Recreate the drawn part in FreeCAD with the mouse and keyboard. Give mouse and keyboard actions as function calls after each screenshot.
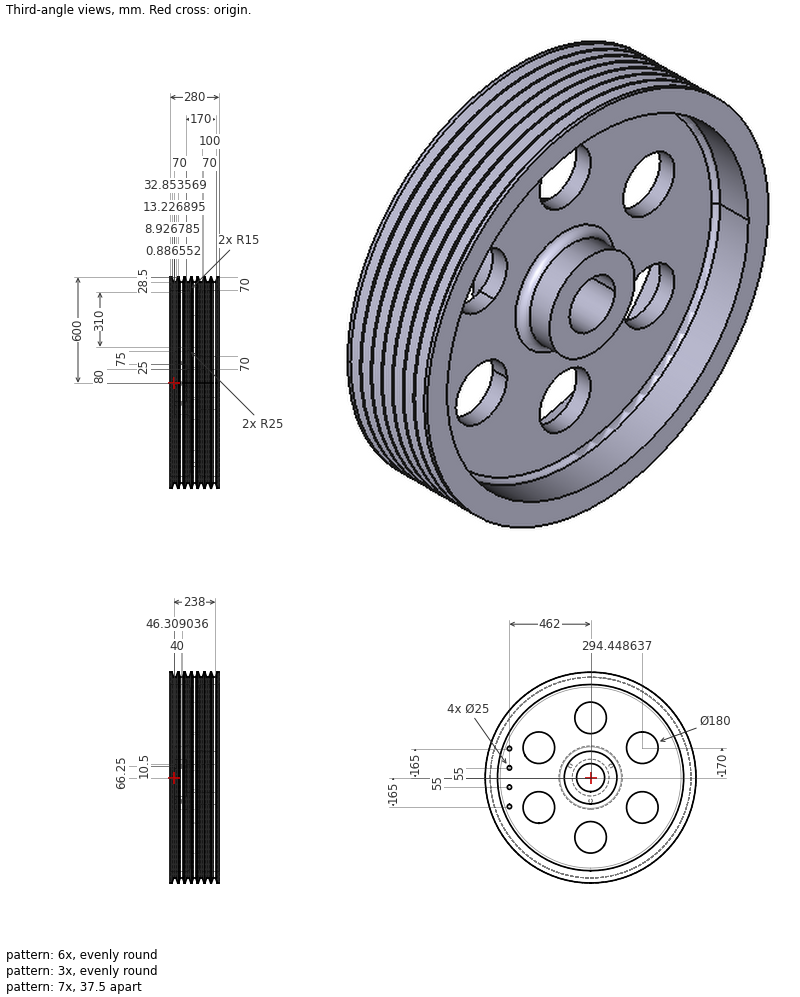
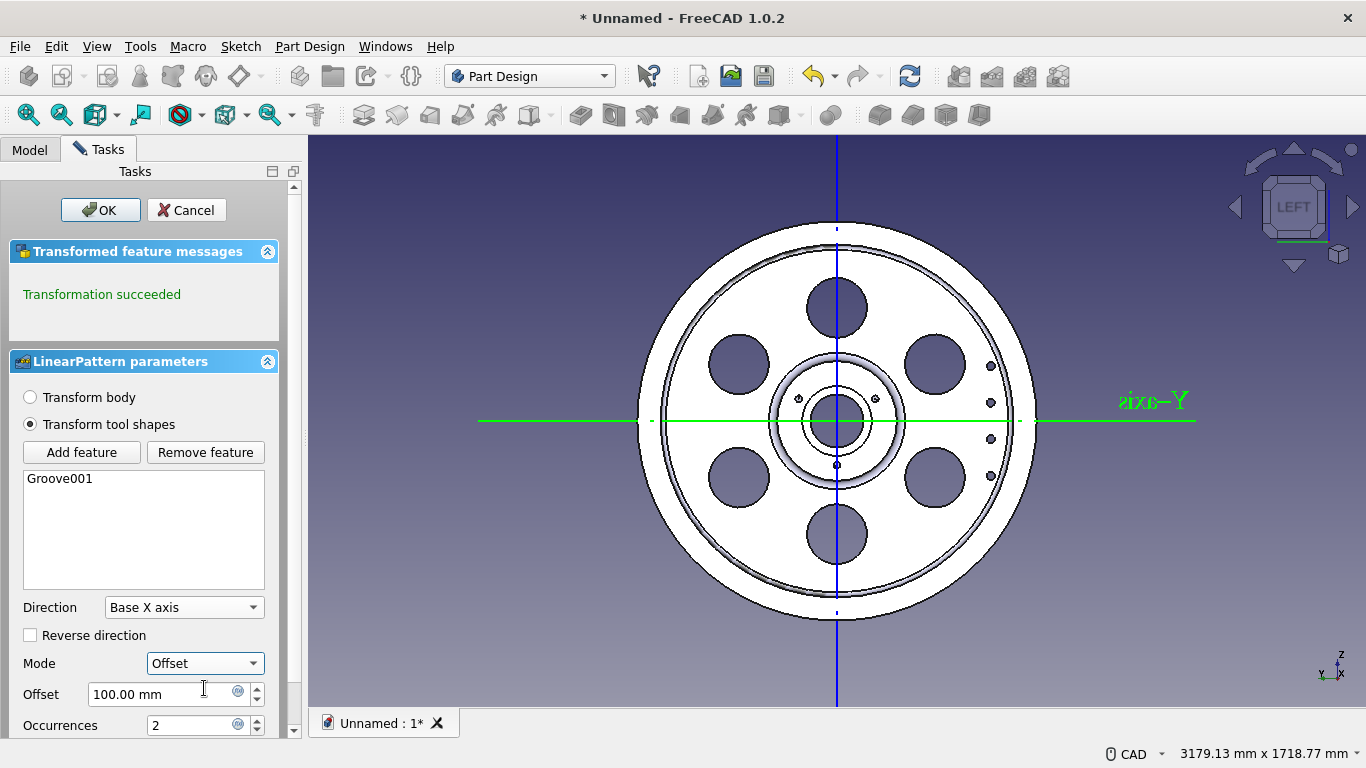
triple_click(170, 694)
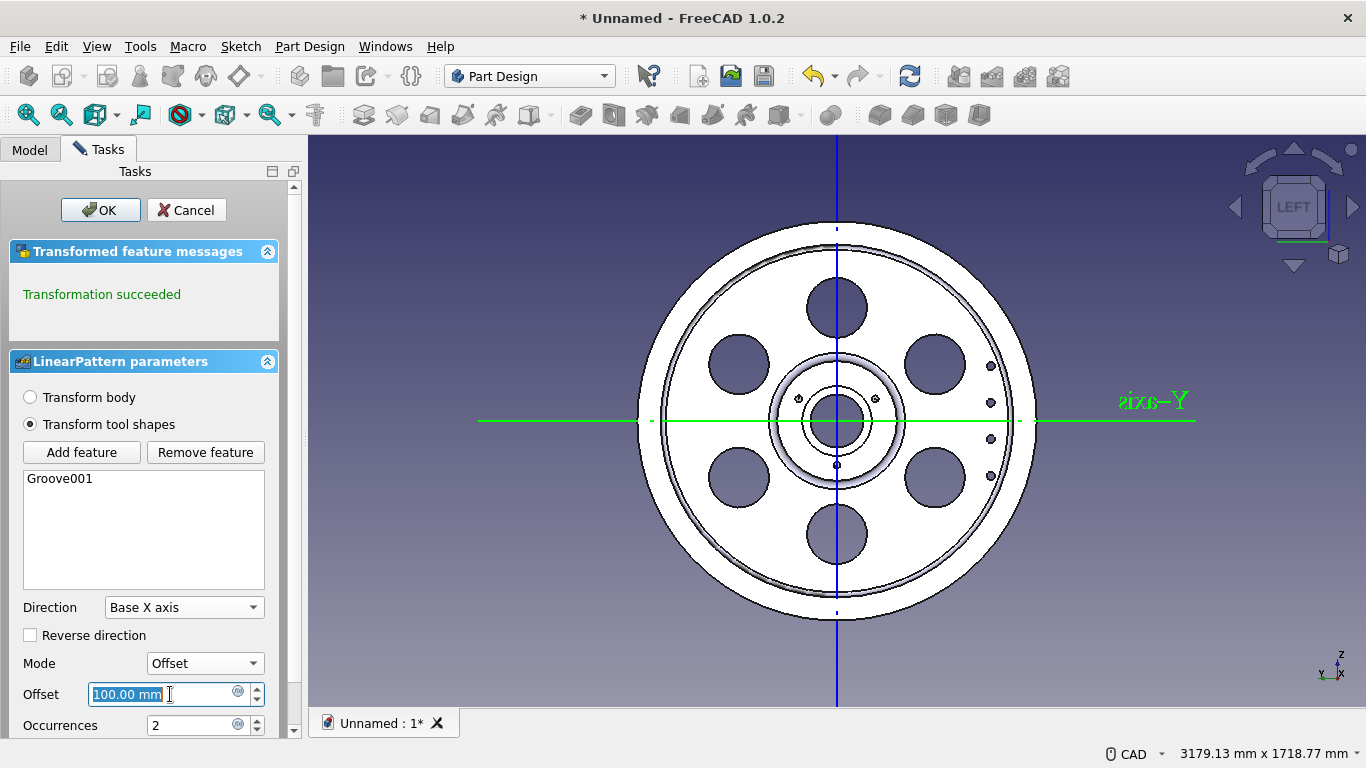
text(37.5)
key(Tab)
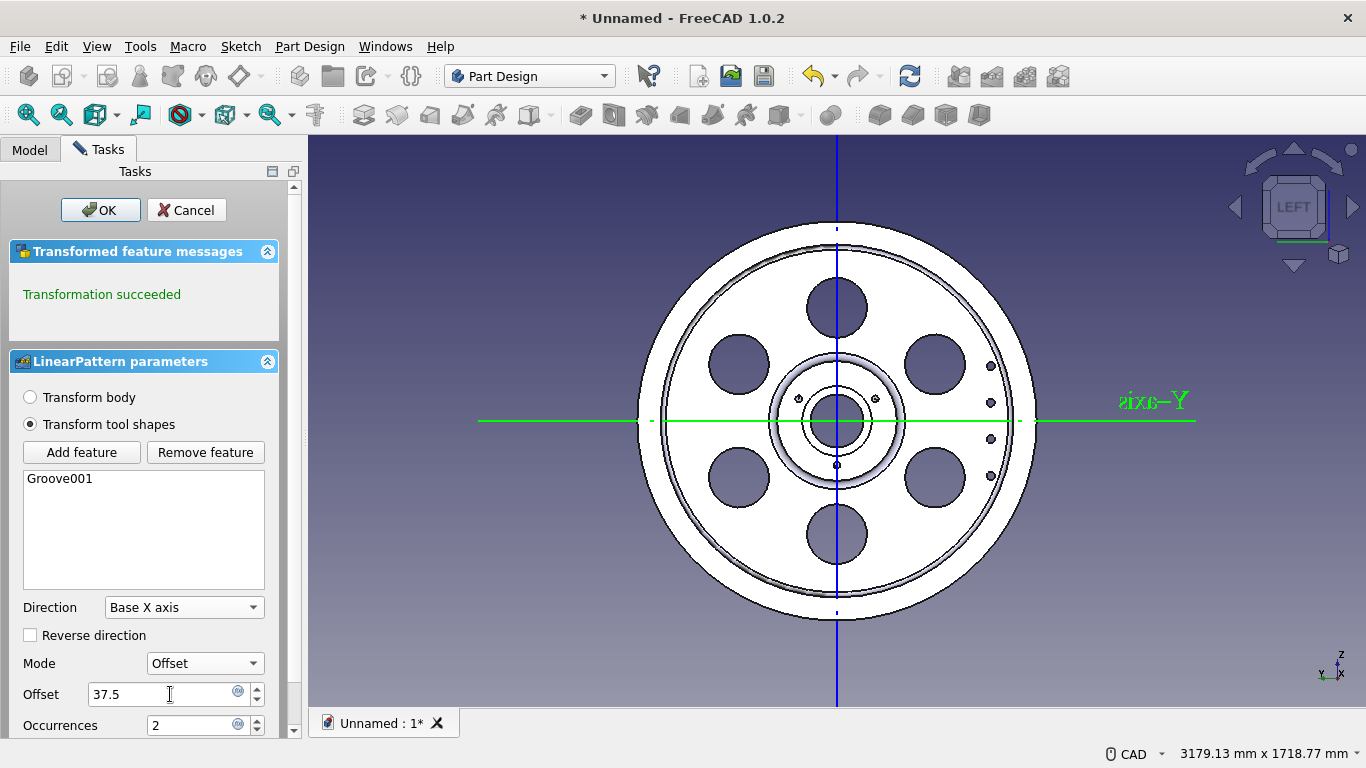
triple_click(199, 726)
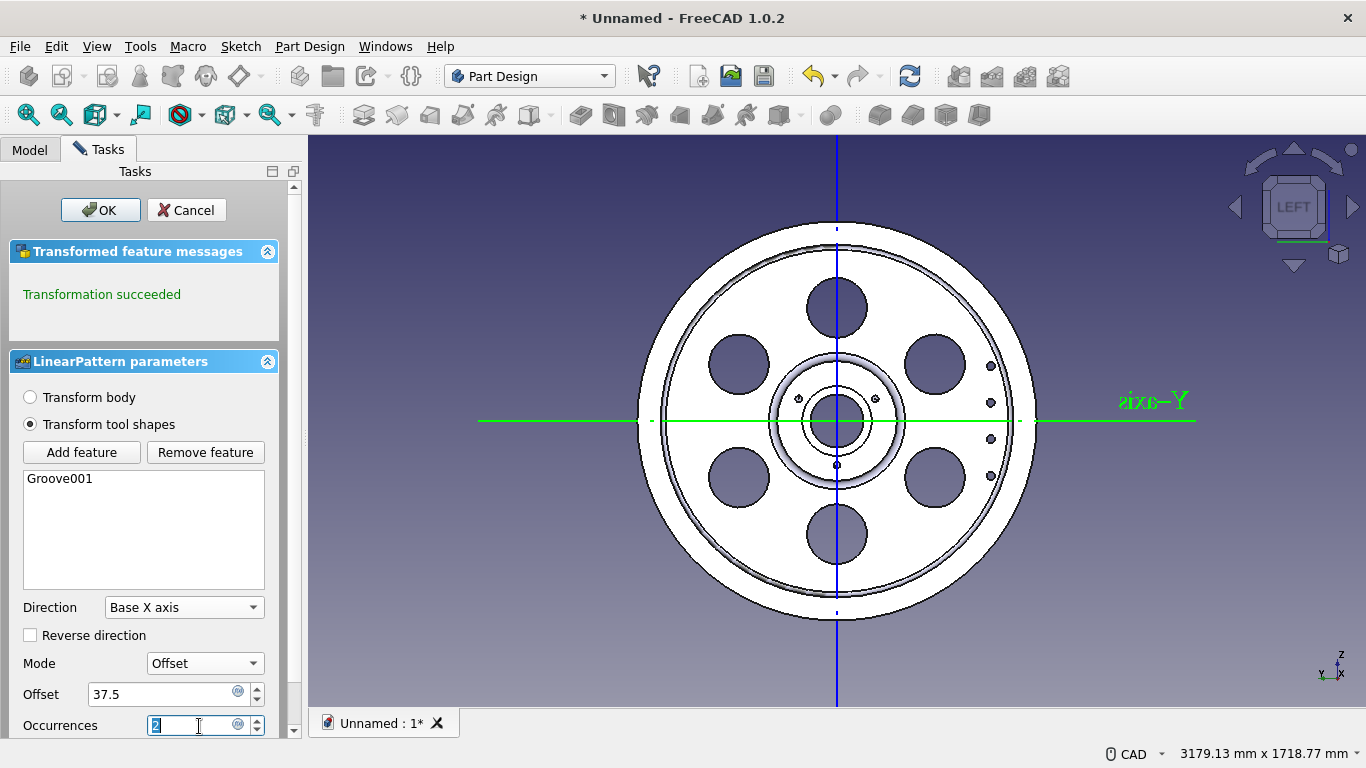
text(7)
key(Tab)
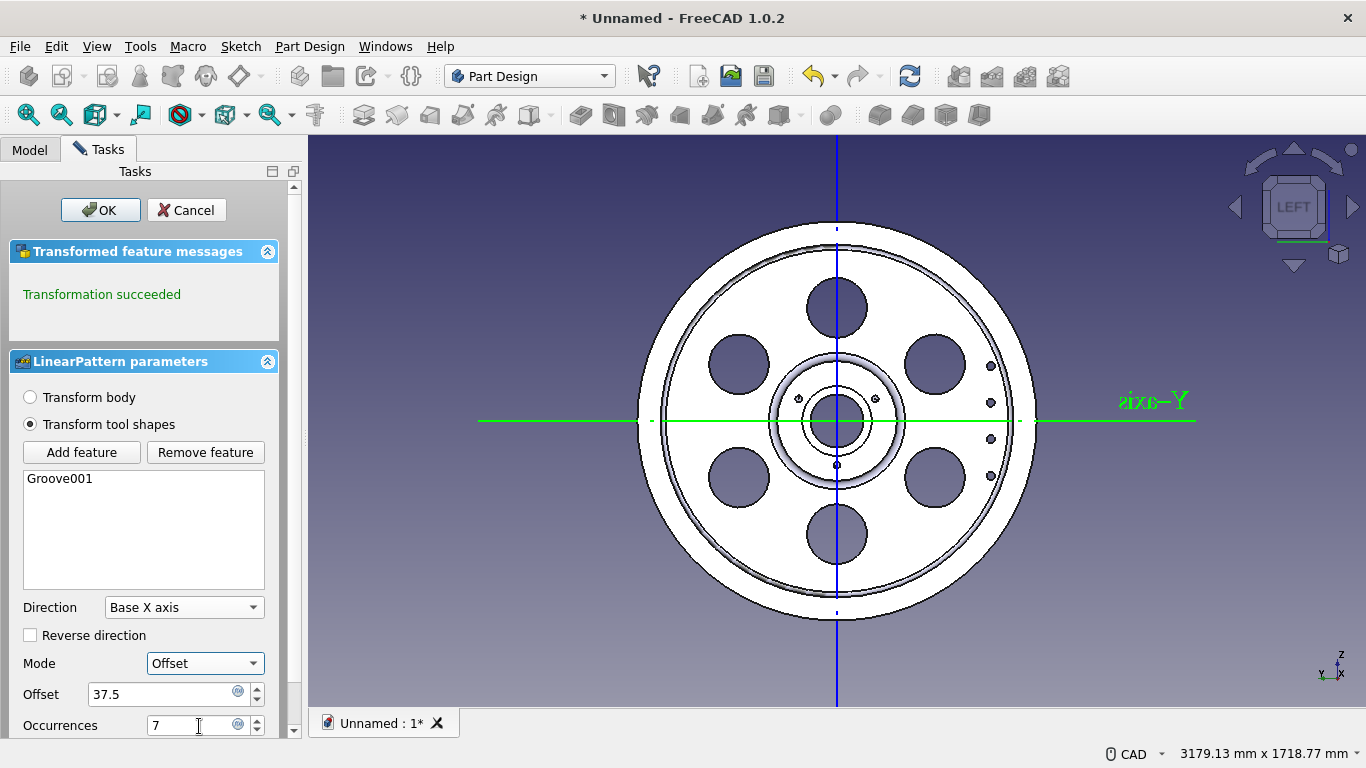
click(101, 210)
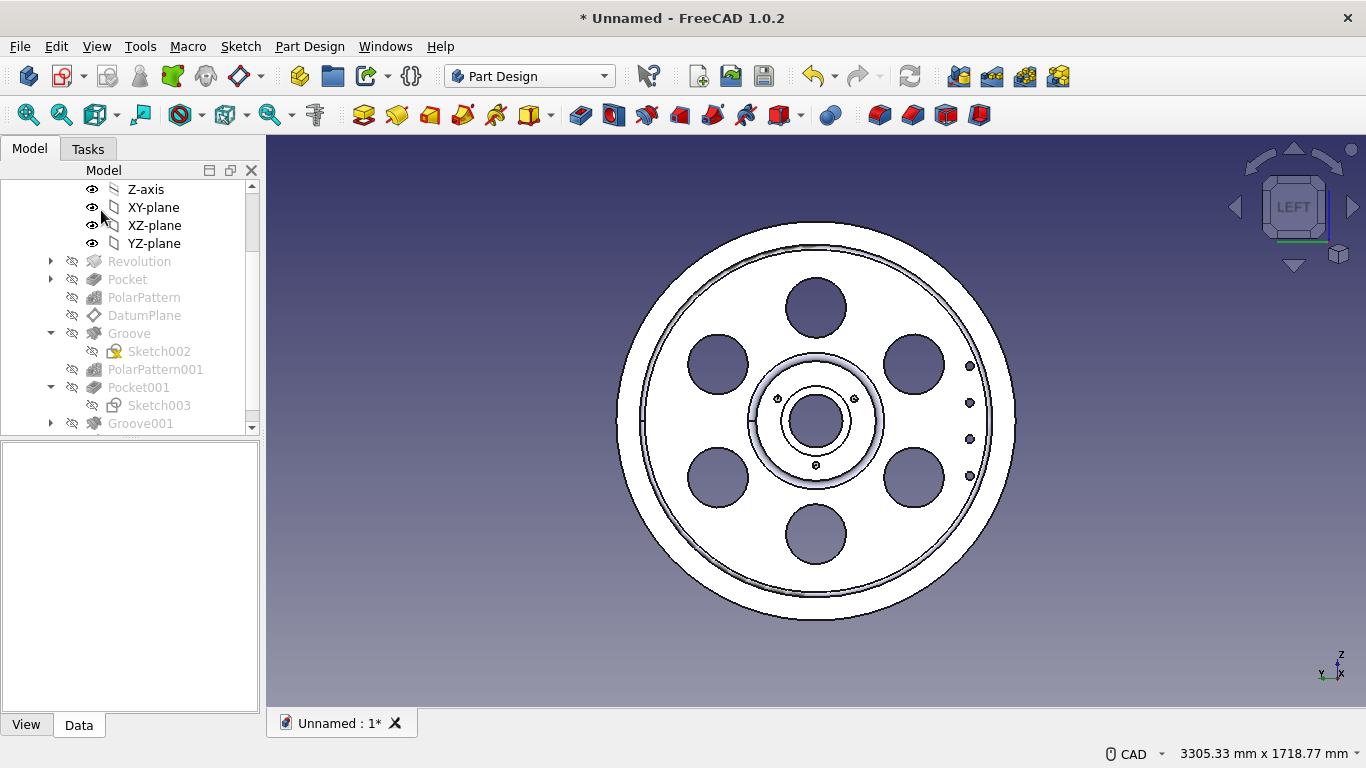
key(0)